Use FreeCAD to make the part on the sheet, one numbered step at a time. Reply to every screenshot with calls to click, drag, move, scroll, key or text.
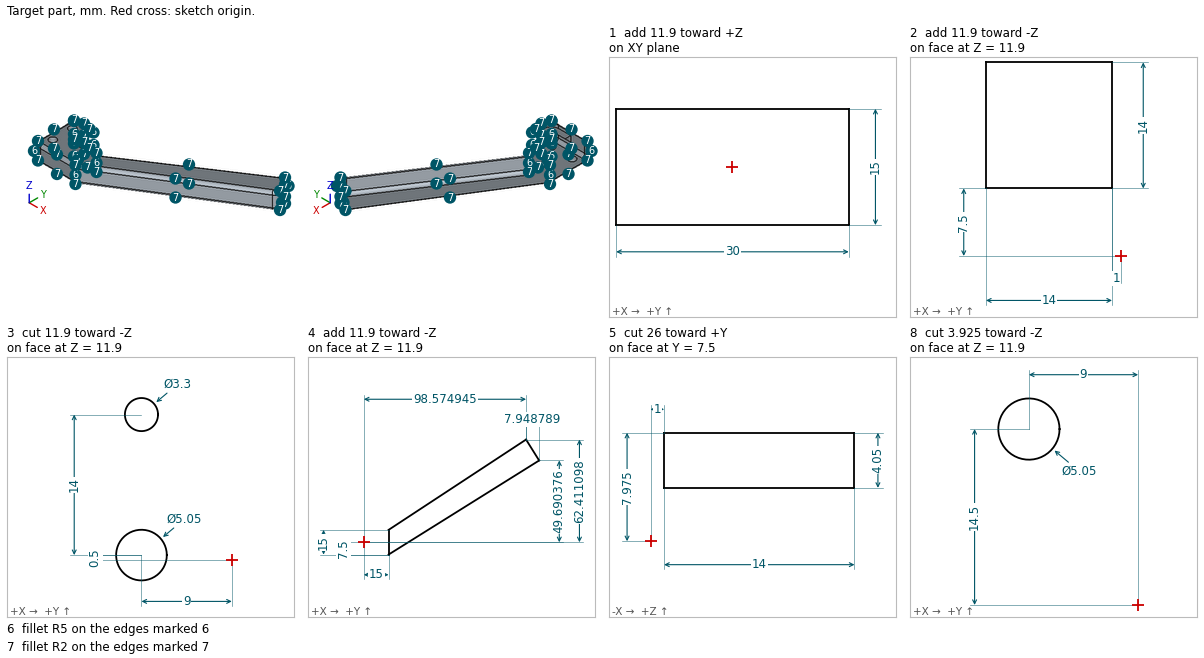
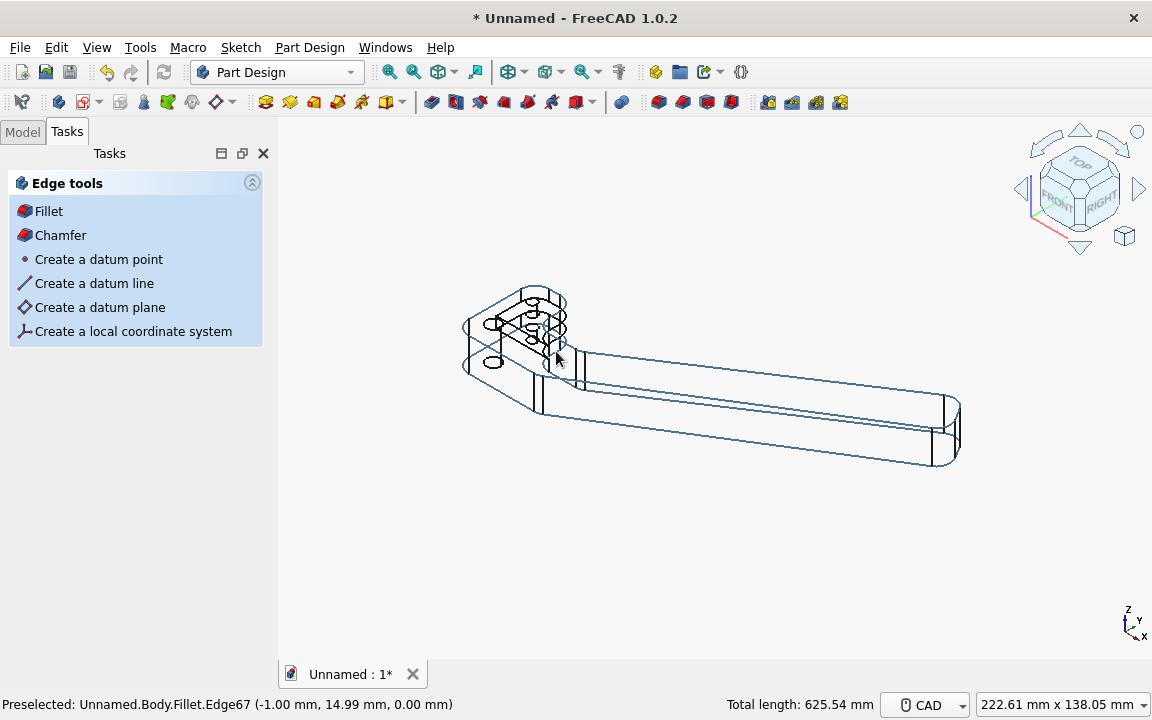
key(v)
key(1)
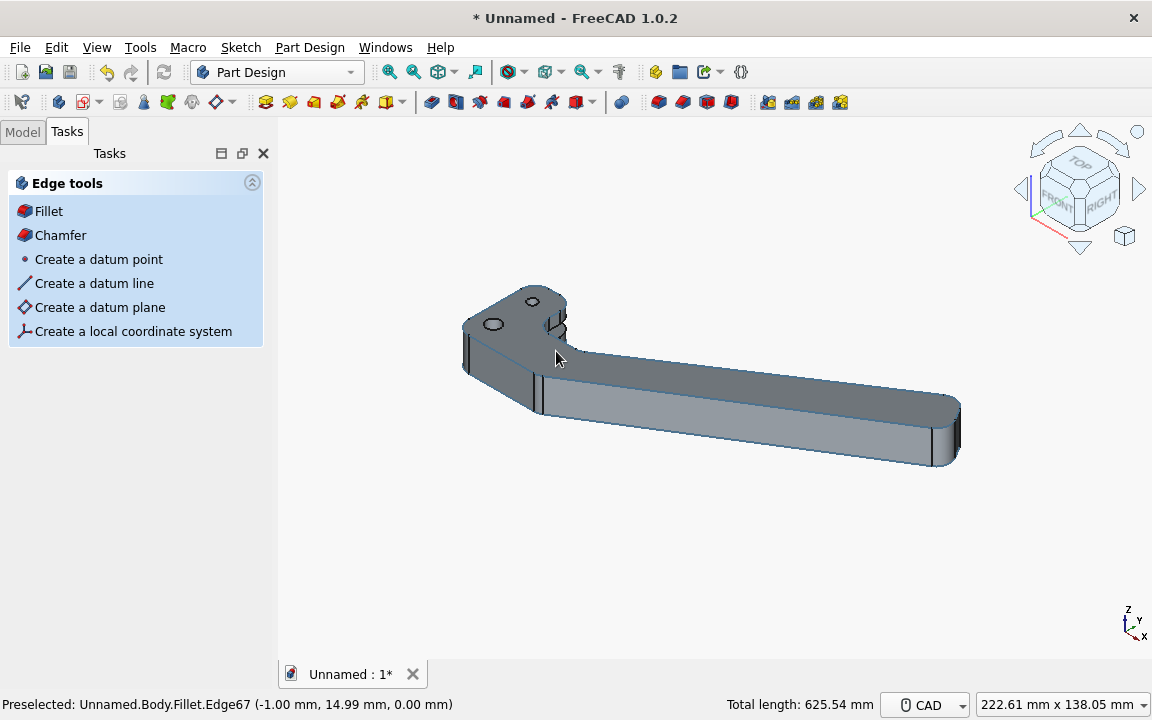
click(660, 102)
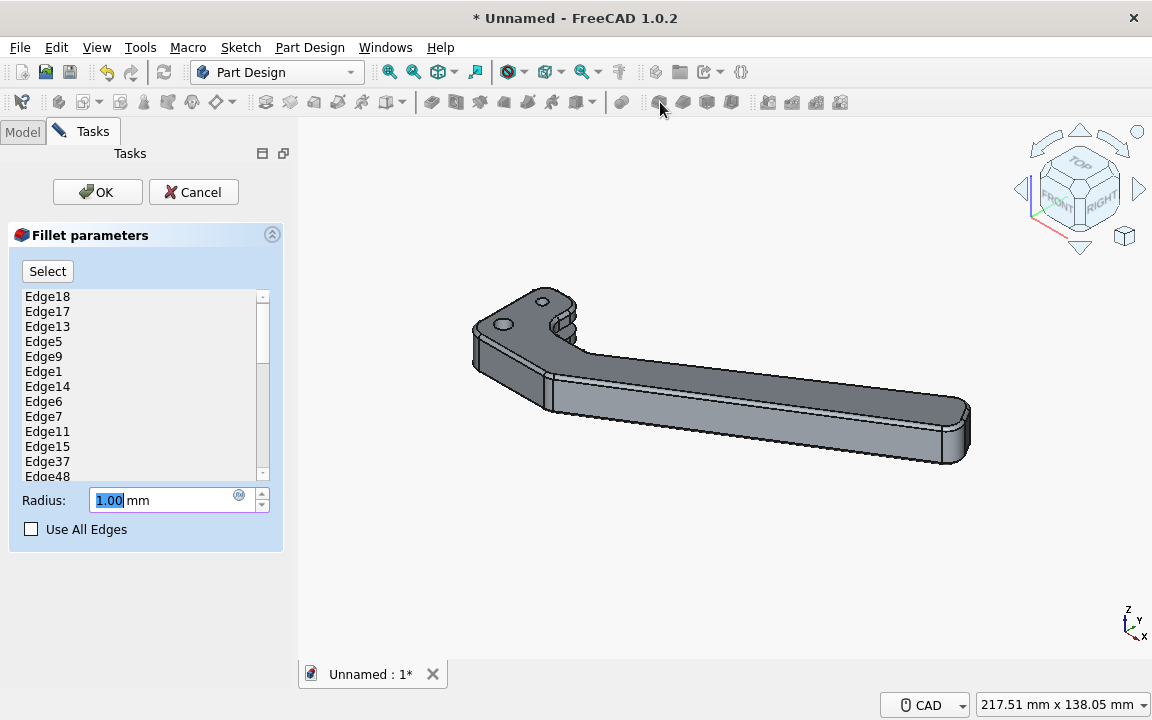
text(2)
key(Tab)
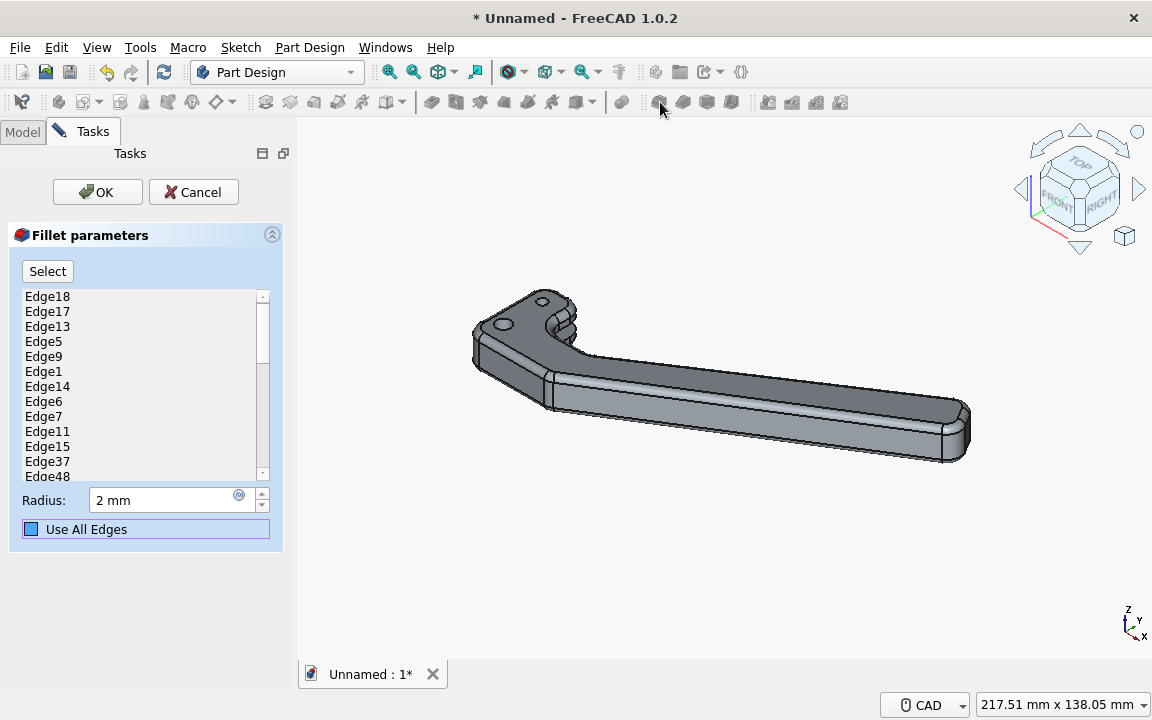
click(98, 192)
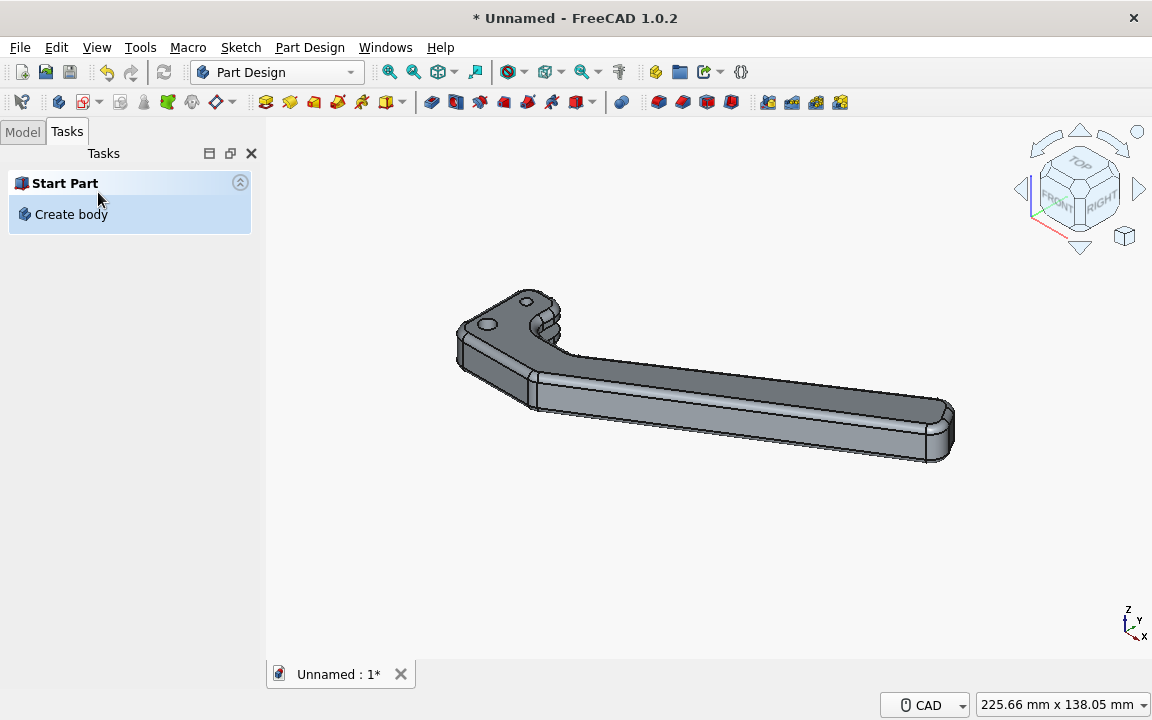
click(541, 359)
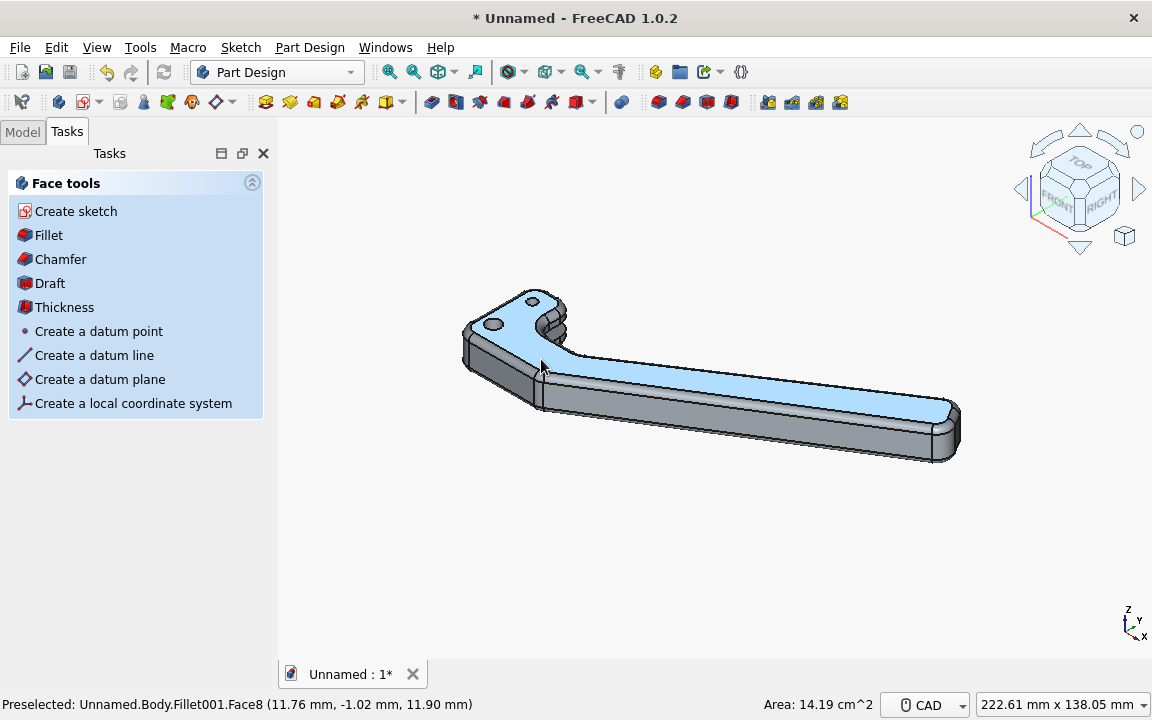
click(84, 102)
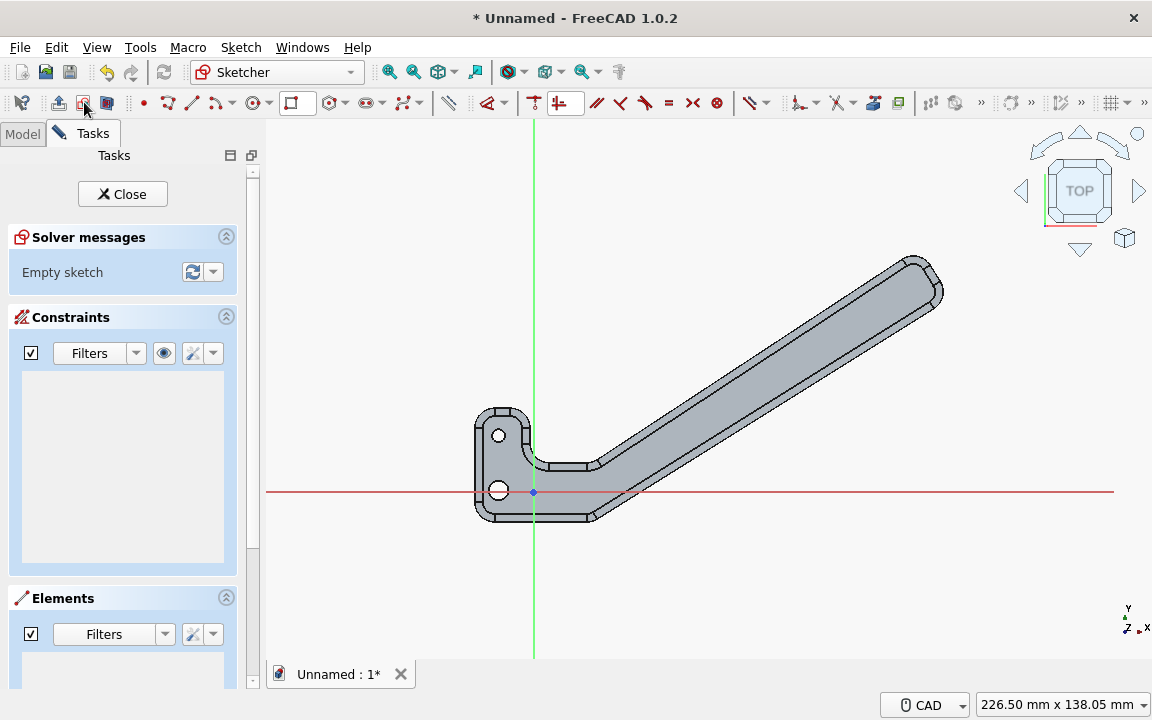
scroll(489, 439, up, 14)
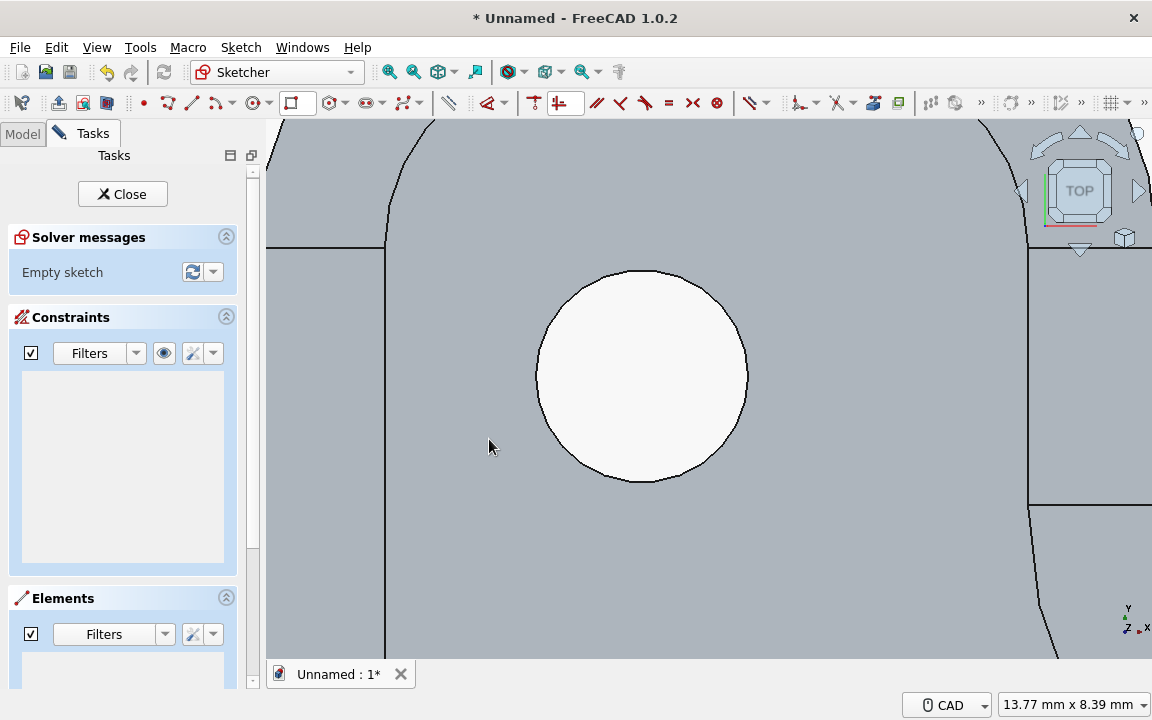
click(254, 104)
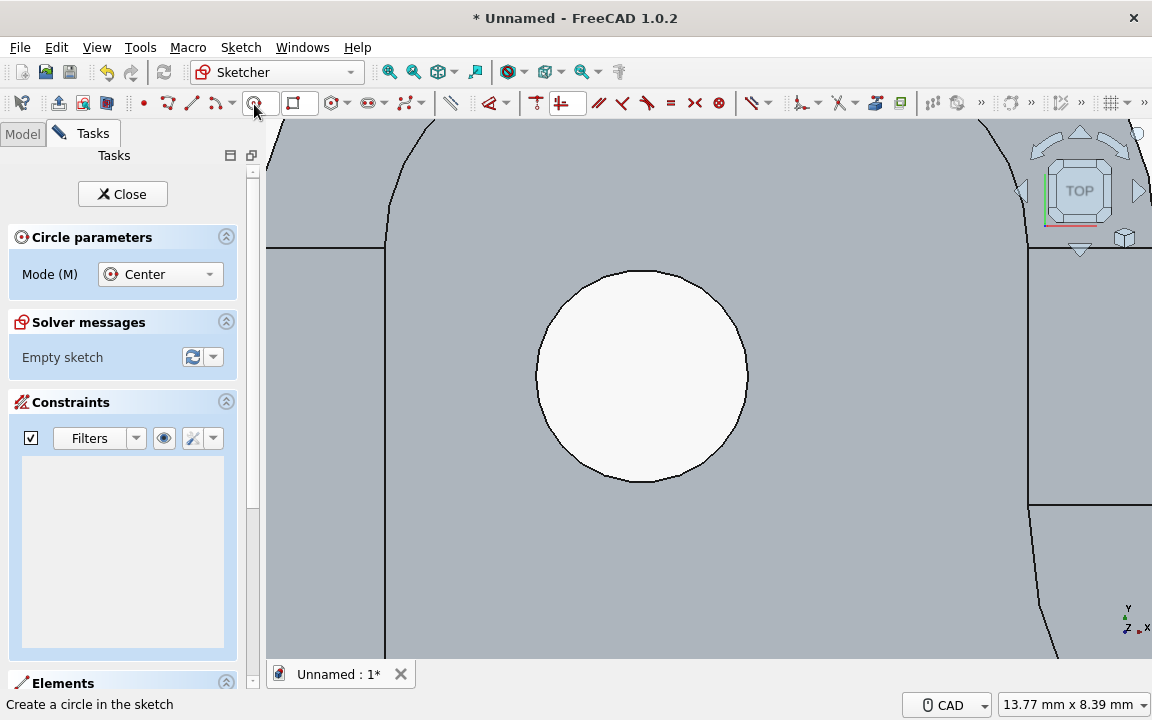
click(642, 376)
move(757, 261)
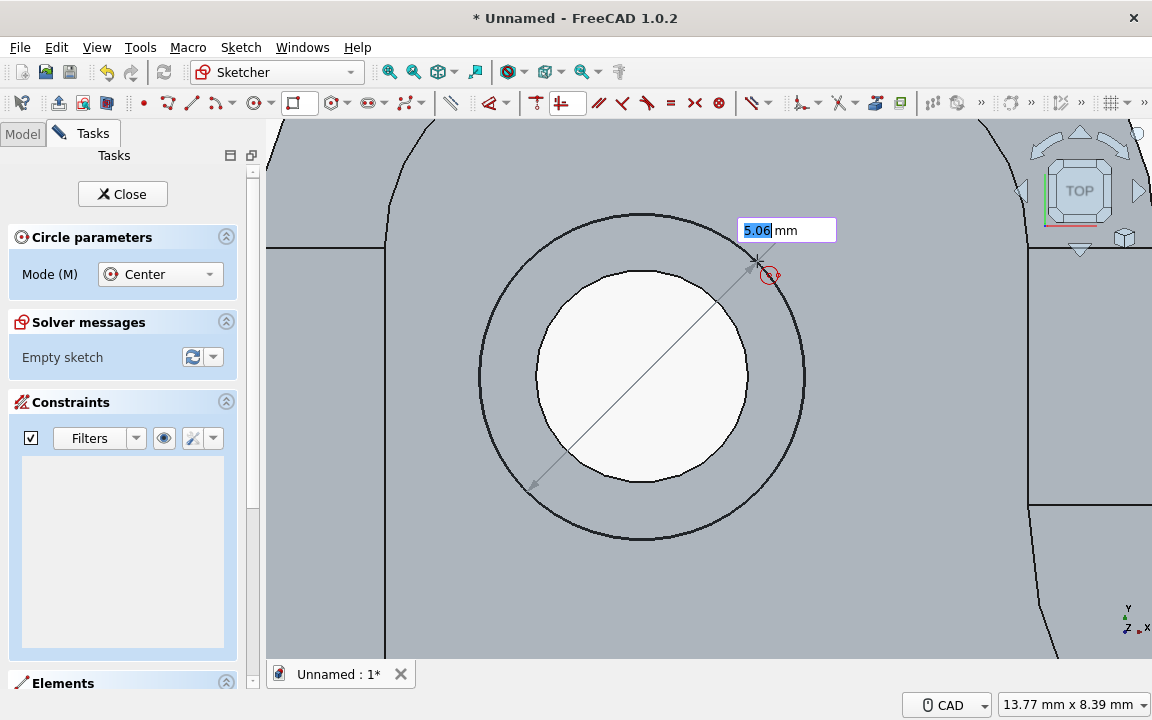
text(5.05)
key(Return)
key(Escape)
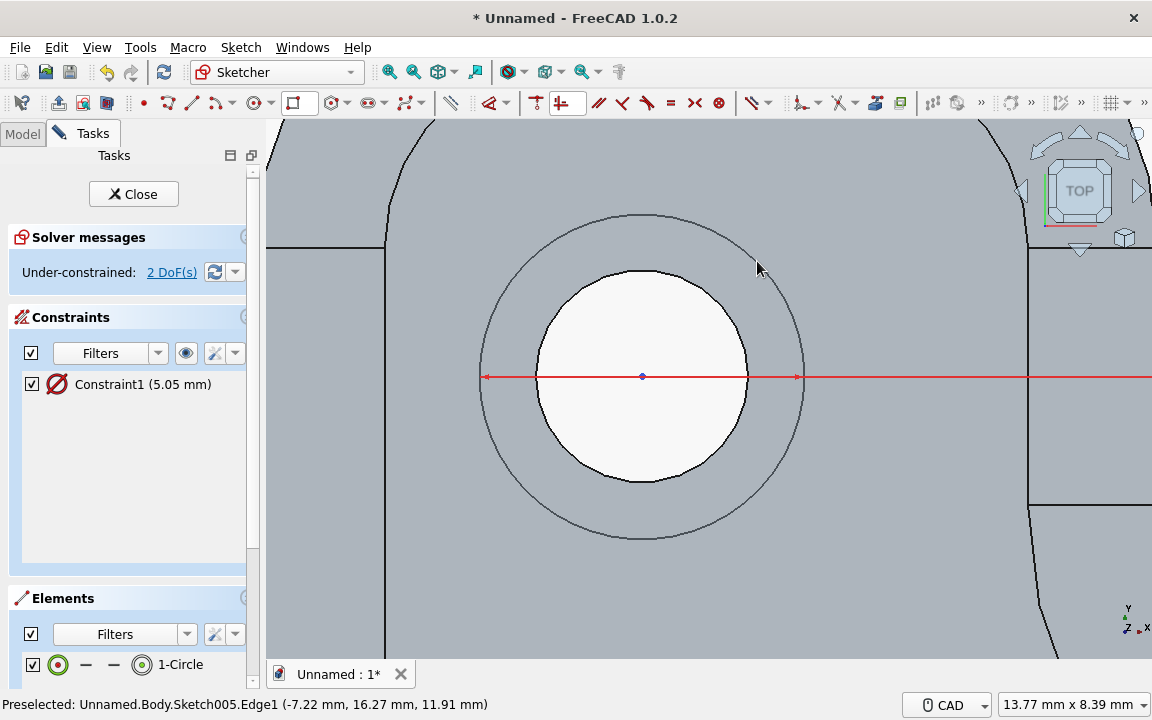
click(490, 104)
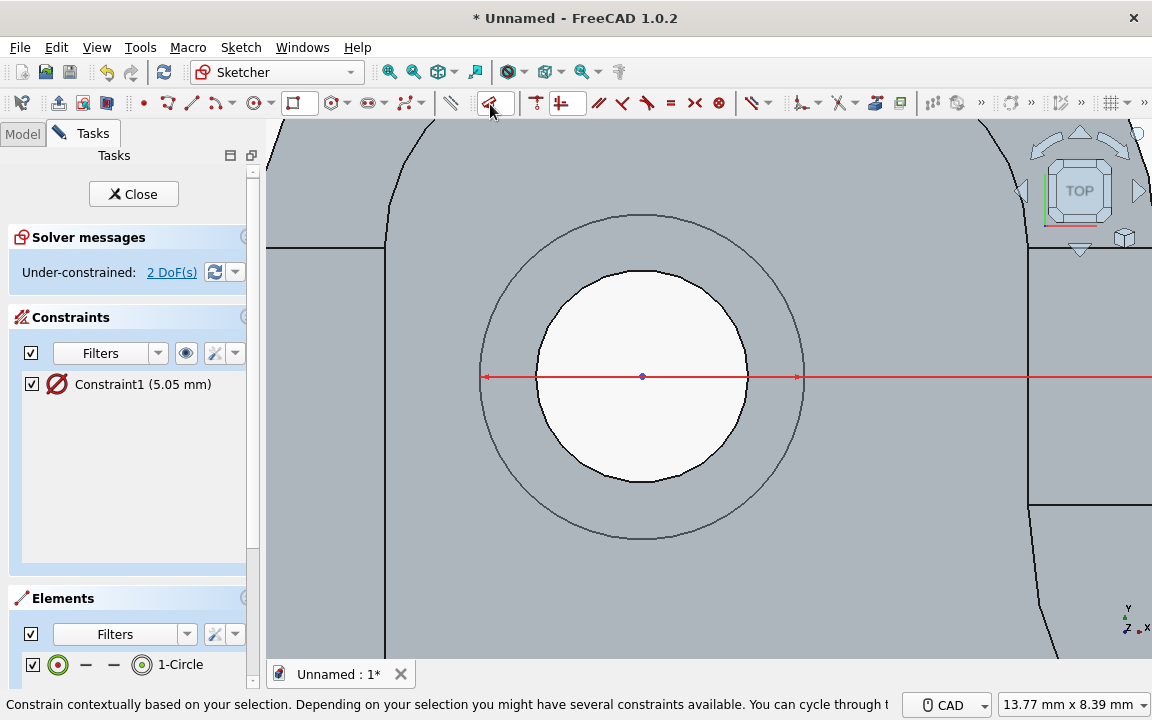
click(642, 377)
click(815, 343)